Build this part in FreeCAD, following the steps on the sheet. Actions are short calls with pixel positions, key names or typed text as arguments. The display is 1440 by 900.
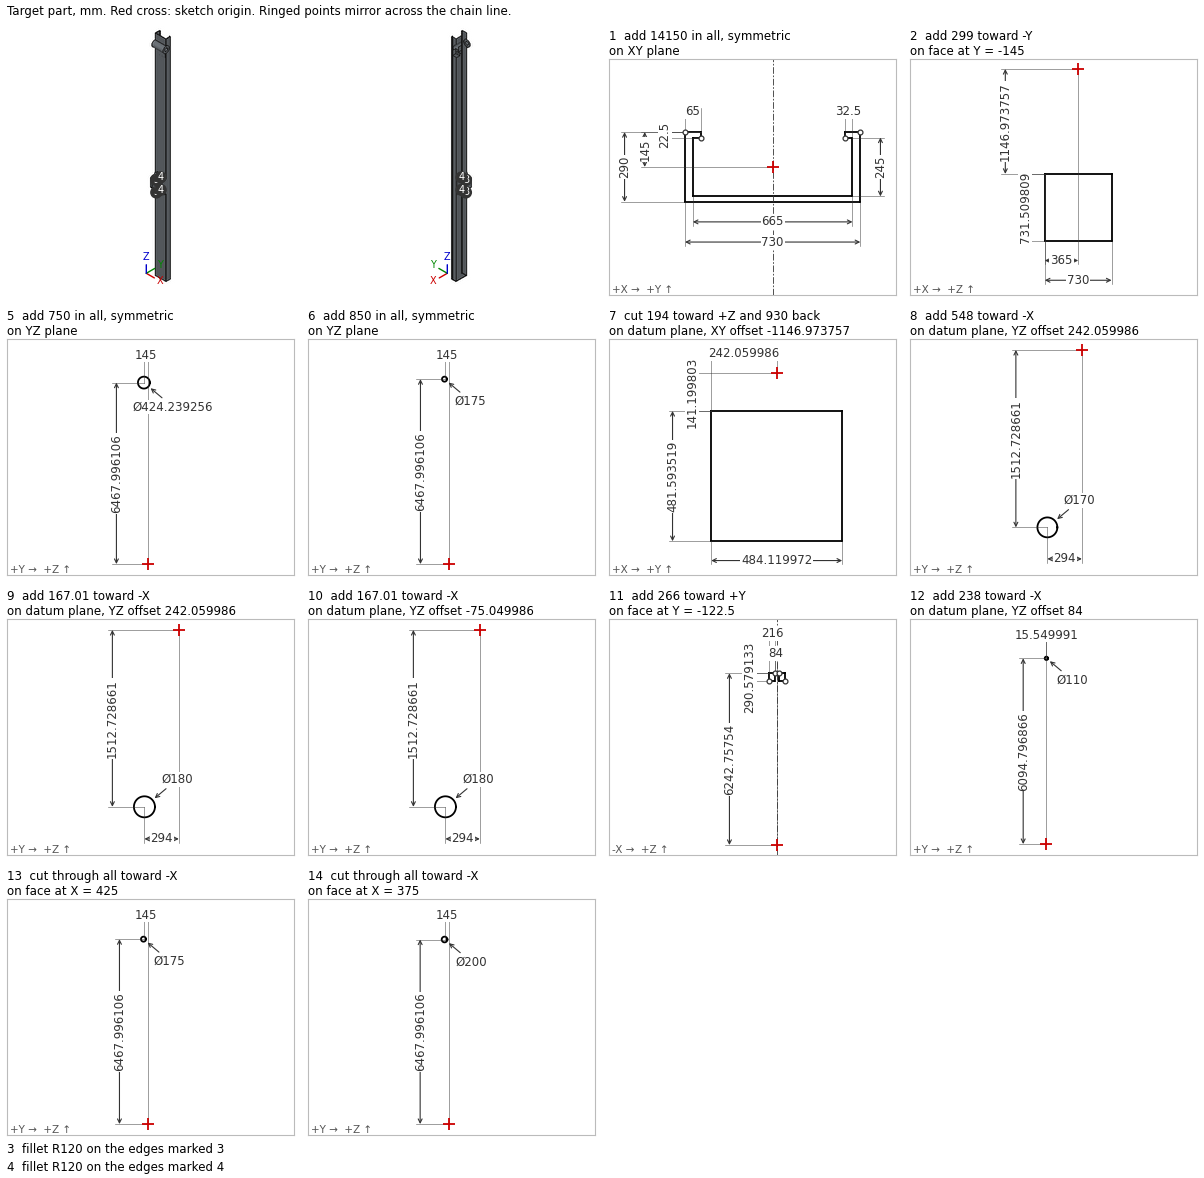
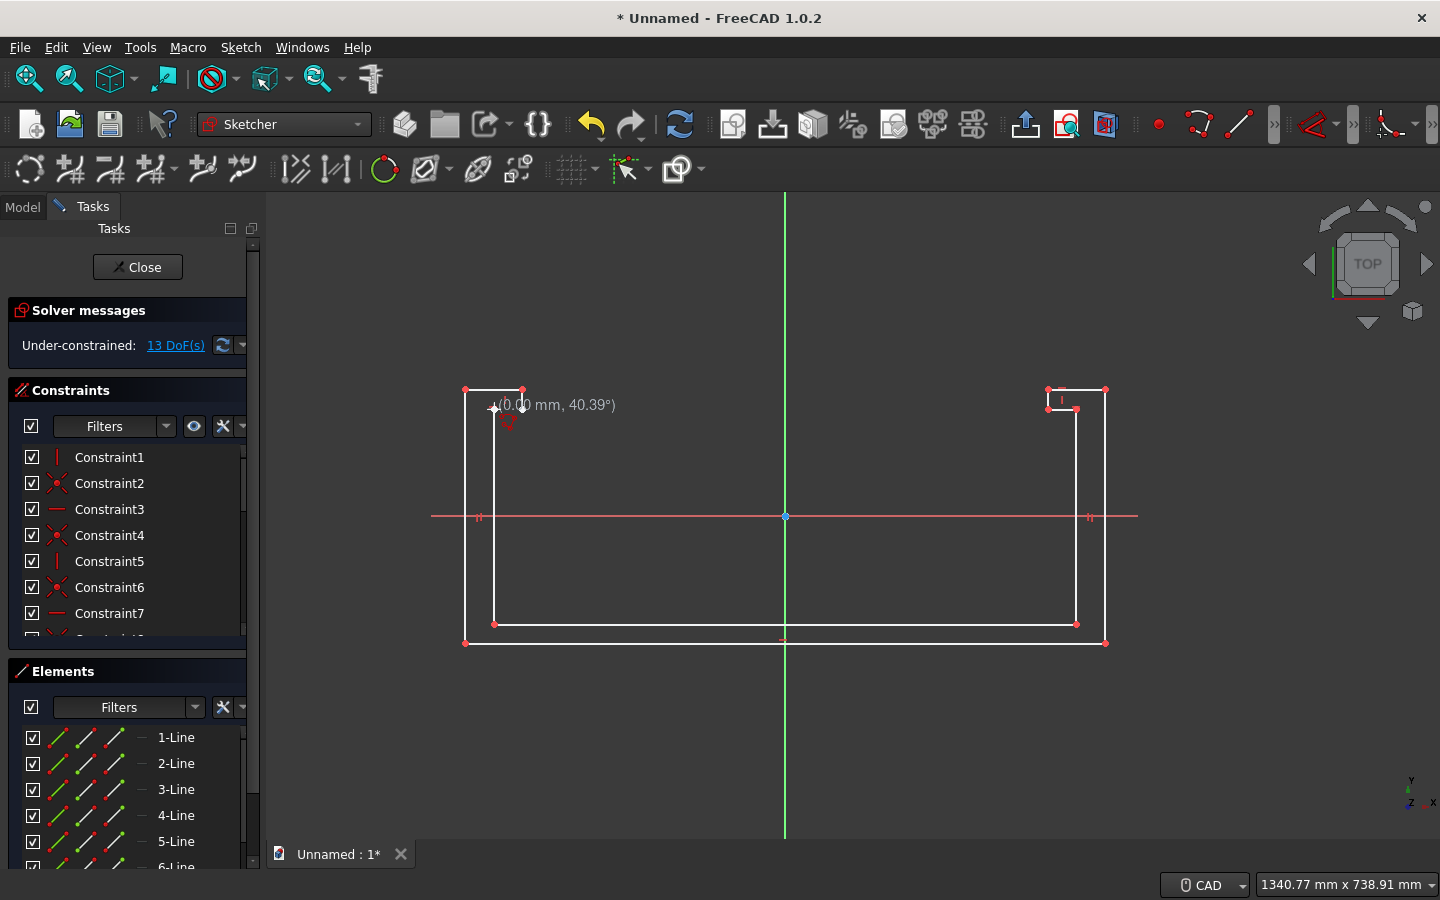
scroll(522, 409, up, 3)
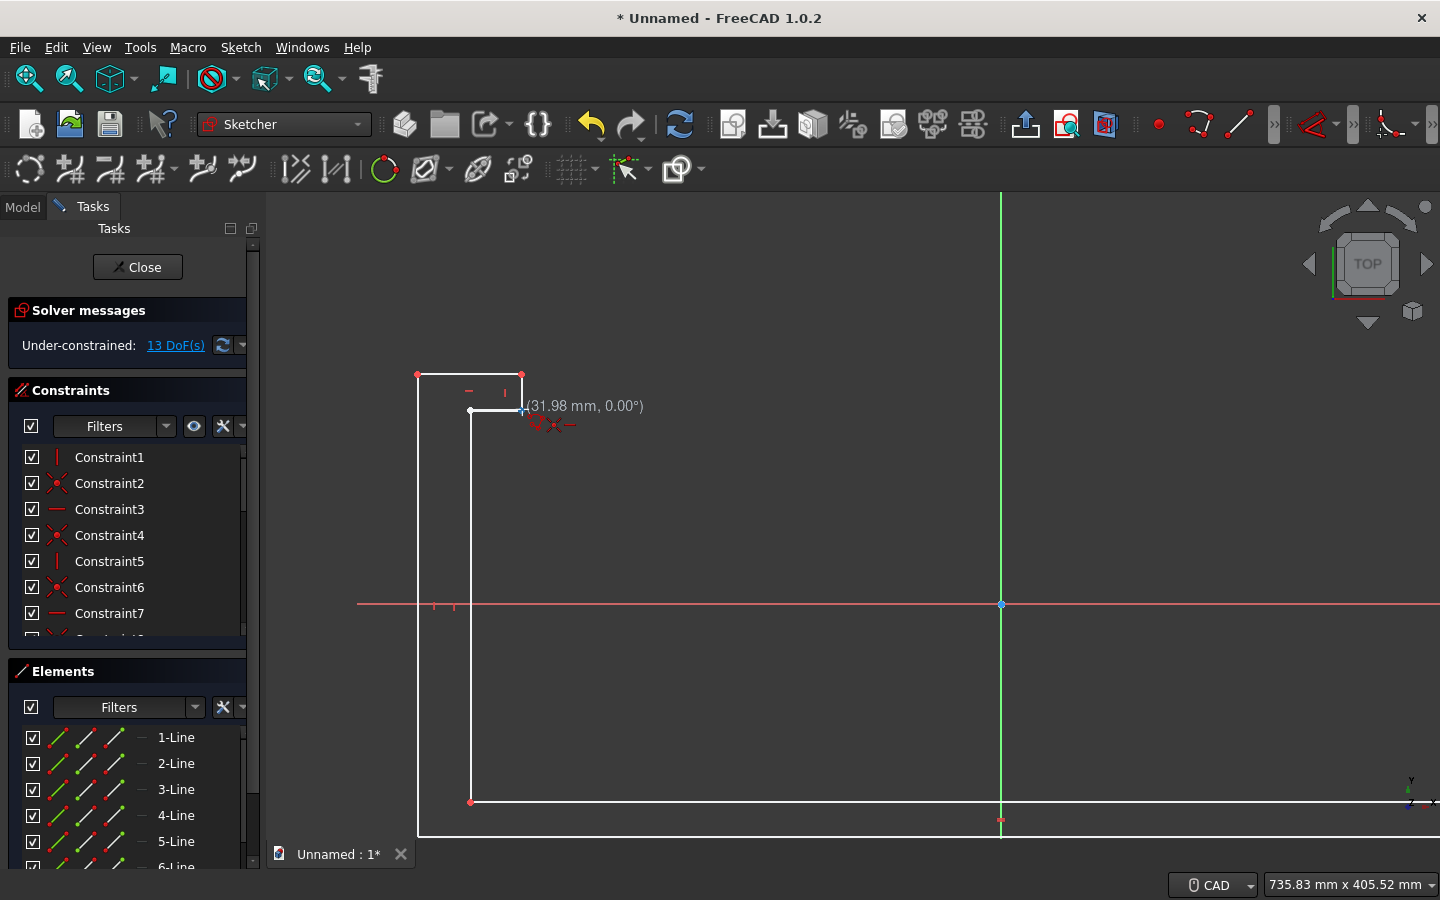
click(522, 411)
key(Escape)
key(Escape)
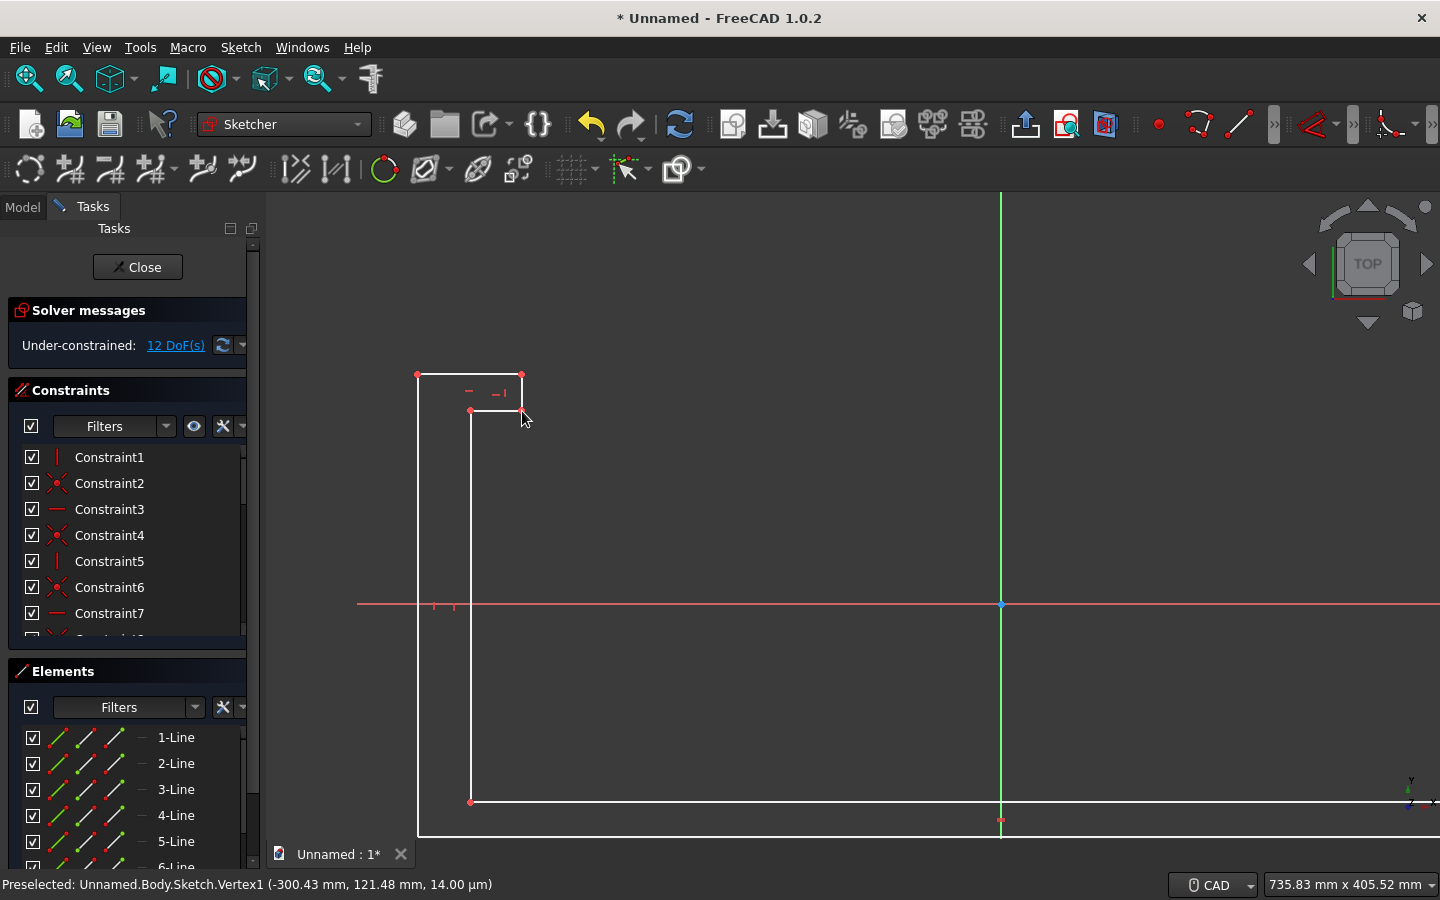
click(418, 374)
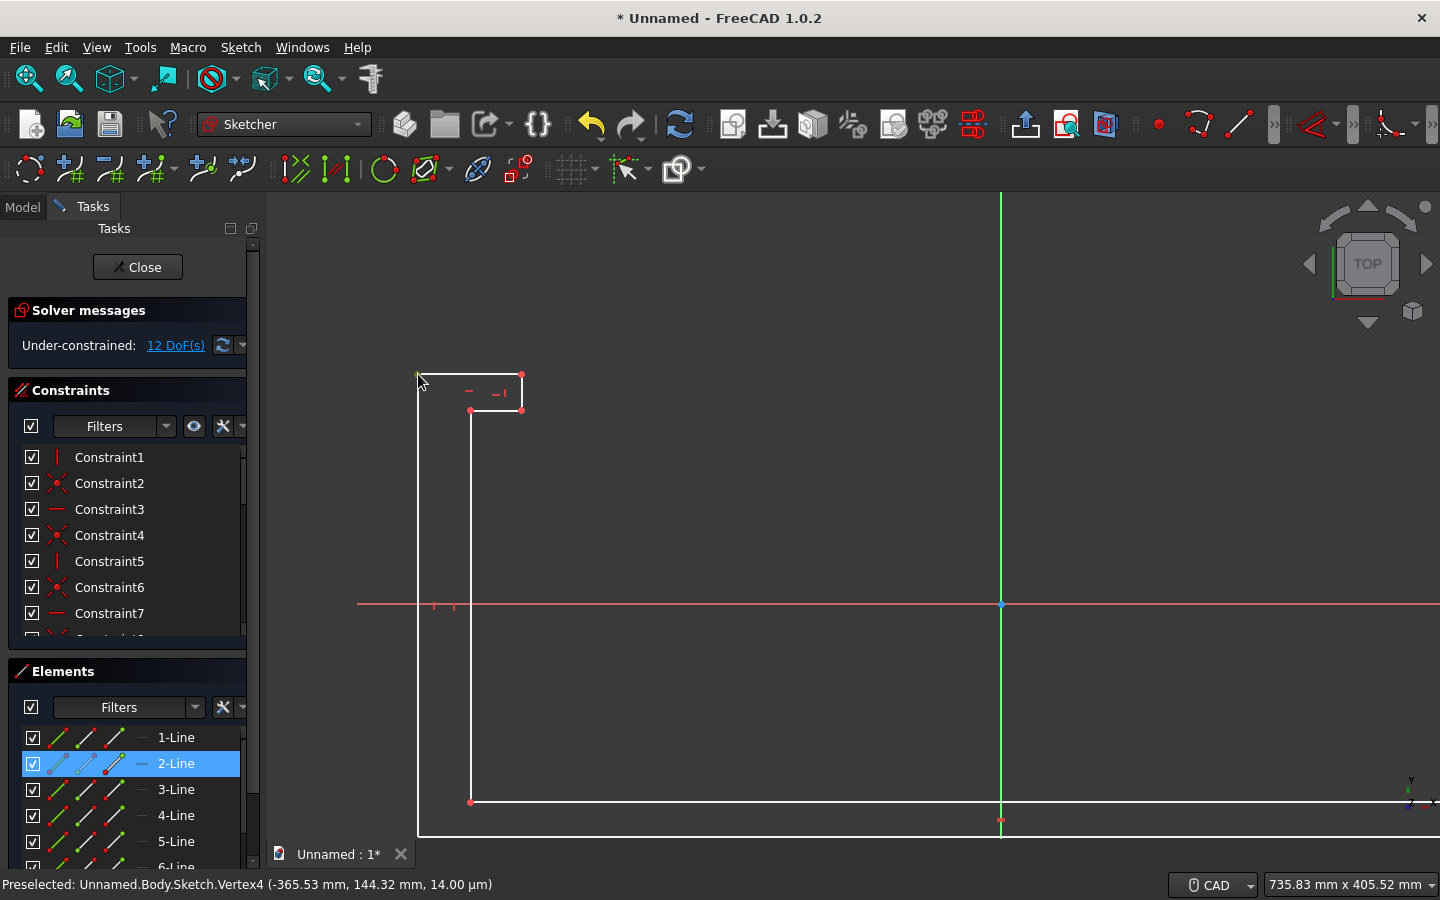
scroll(521, 407, down, 3)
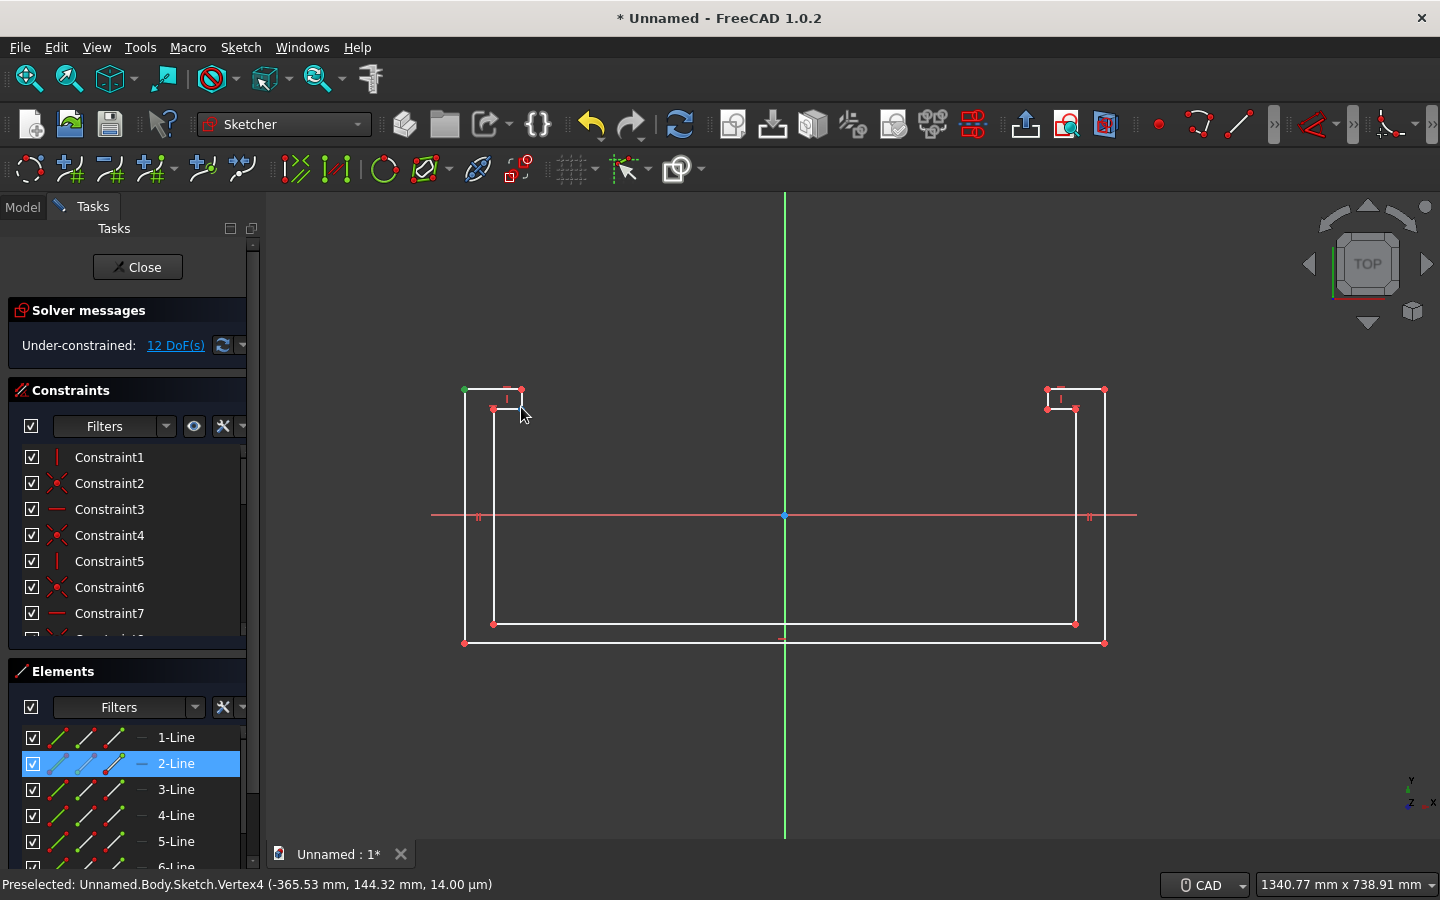
click(1105, 389)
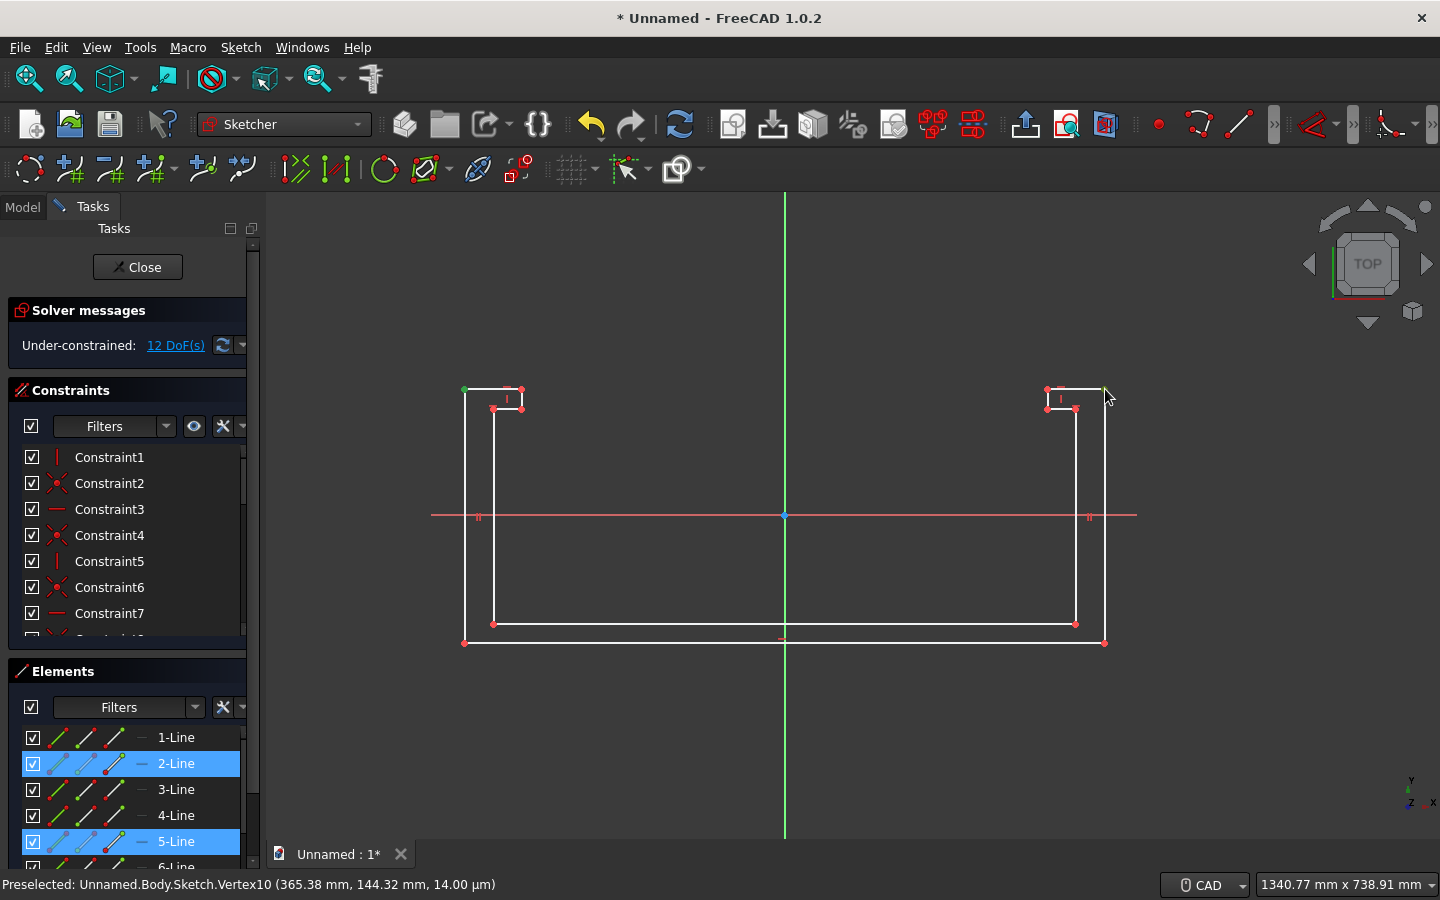
click(785, 769)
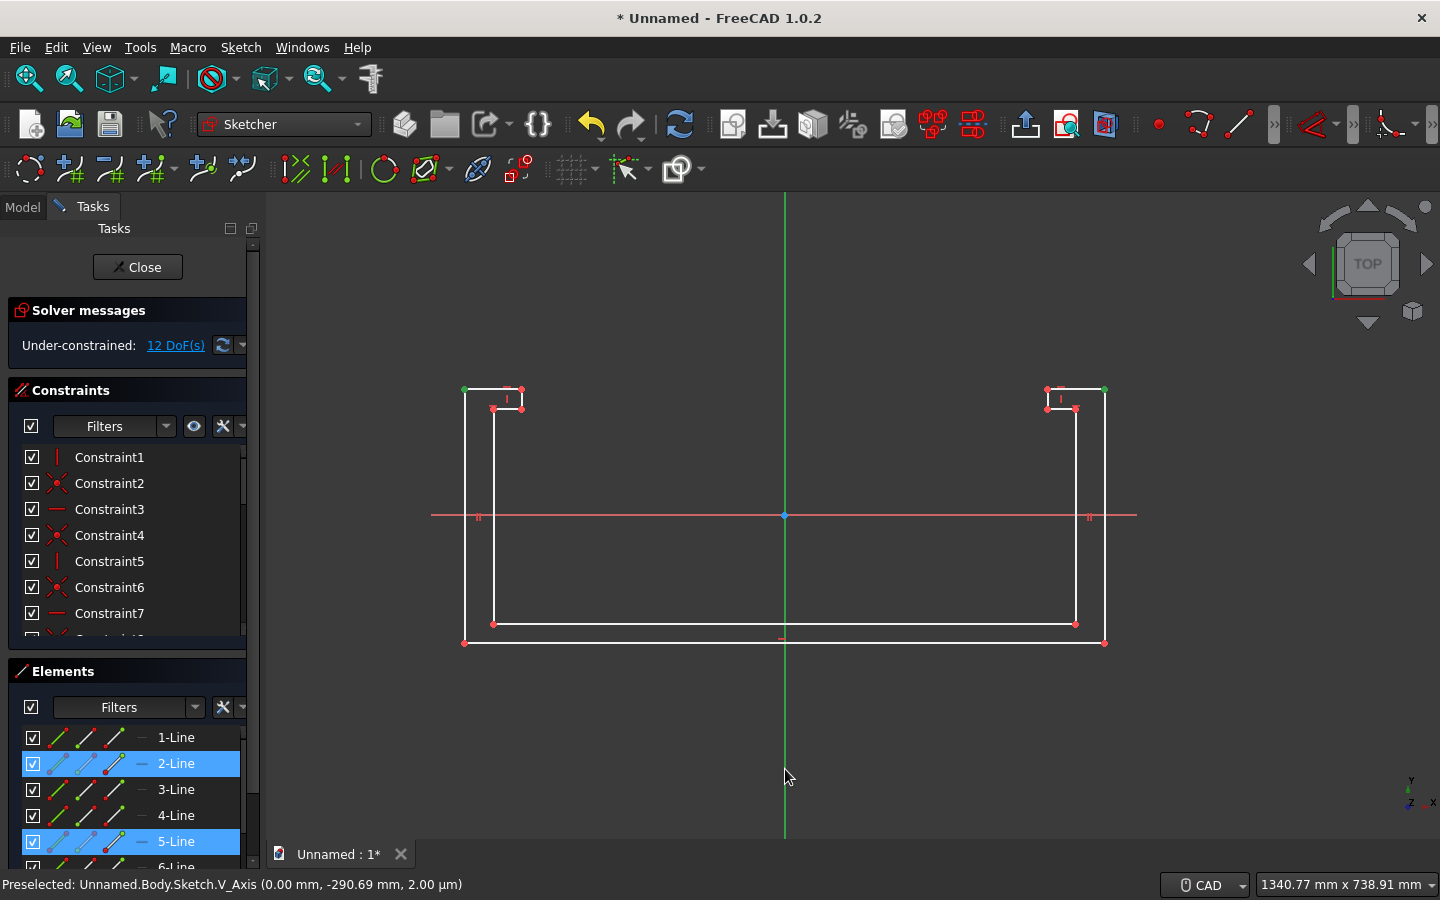
key(s)